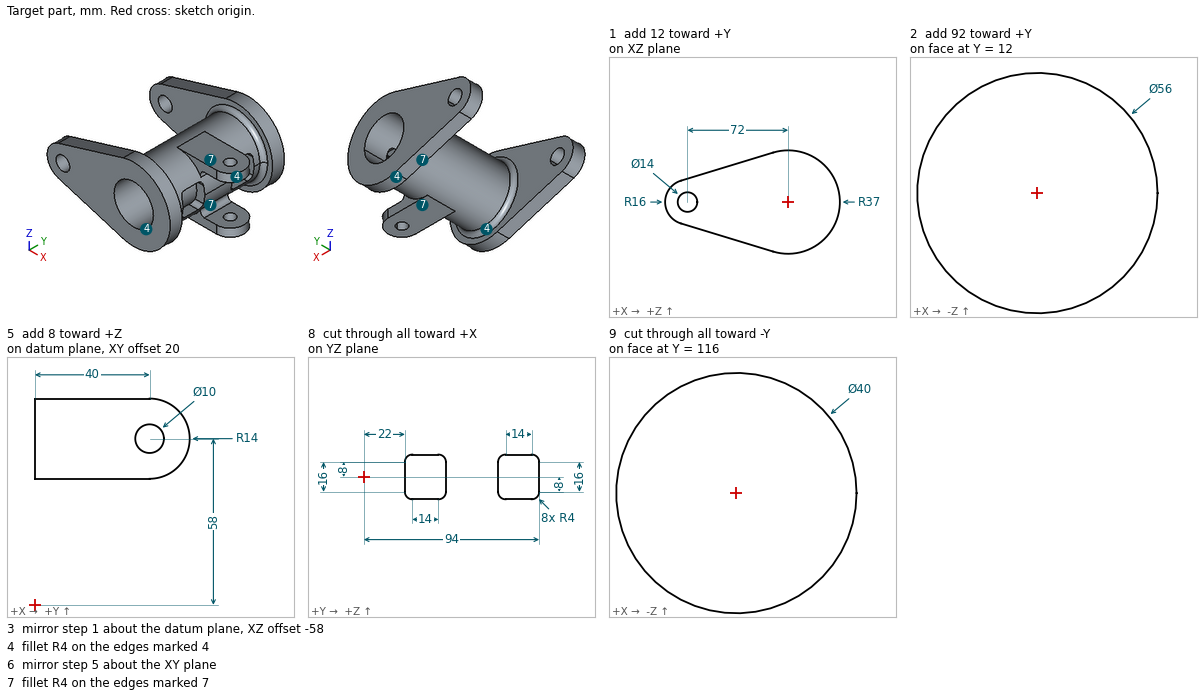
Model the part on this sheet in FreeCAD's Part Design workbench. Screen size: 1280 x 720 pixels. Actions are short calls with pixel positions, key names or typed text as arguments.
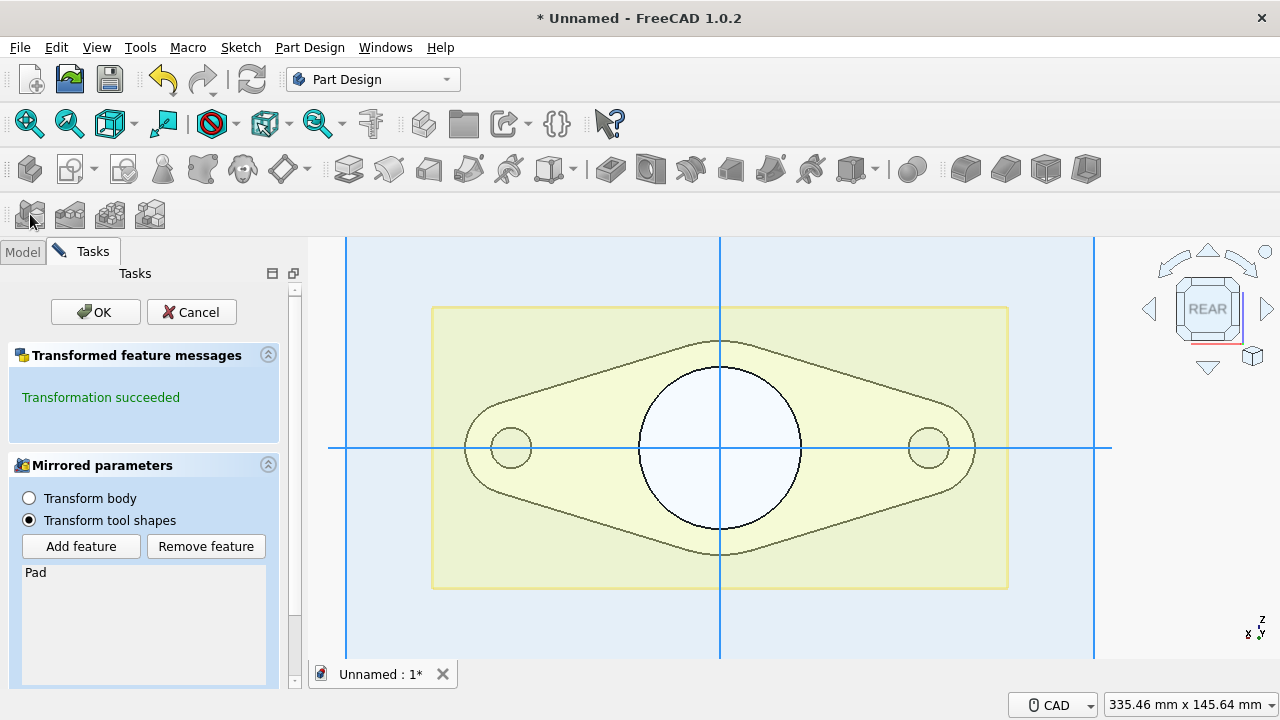
scroll(295, 486, down, 2)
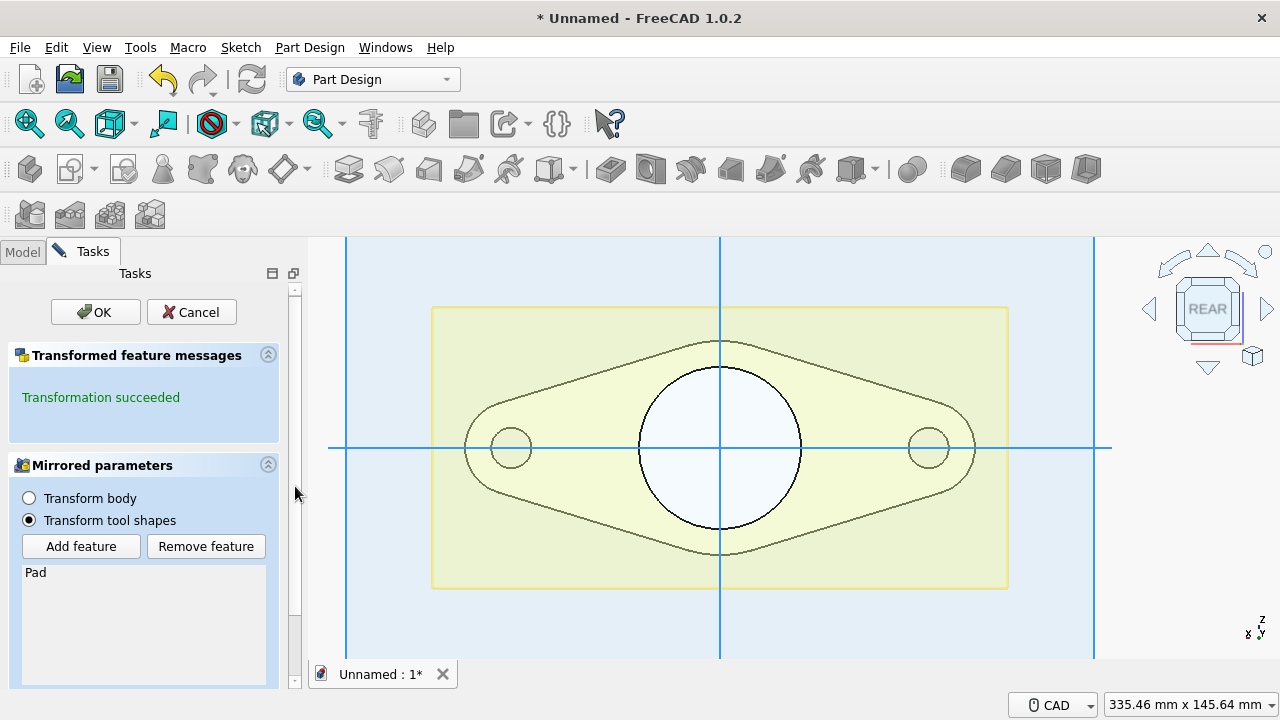
click(184, 628)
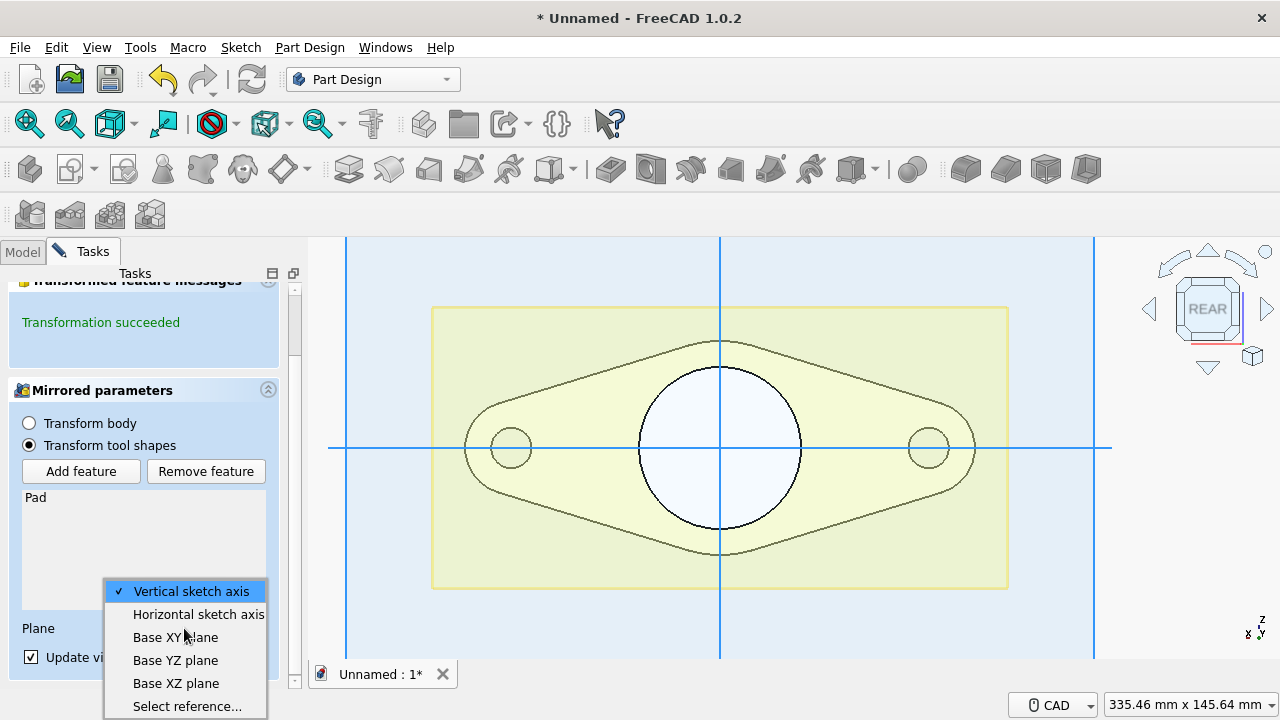
click(184, 706)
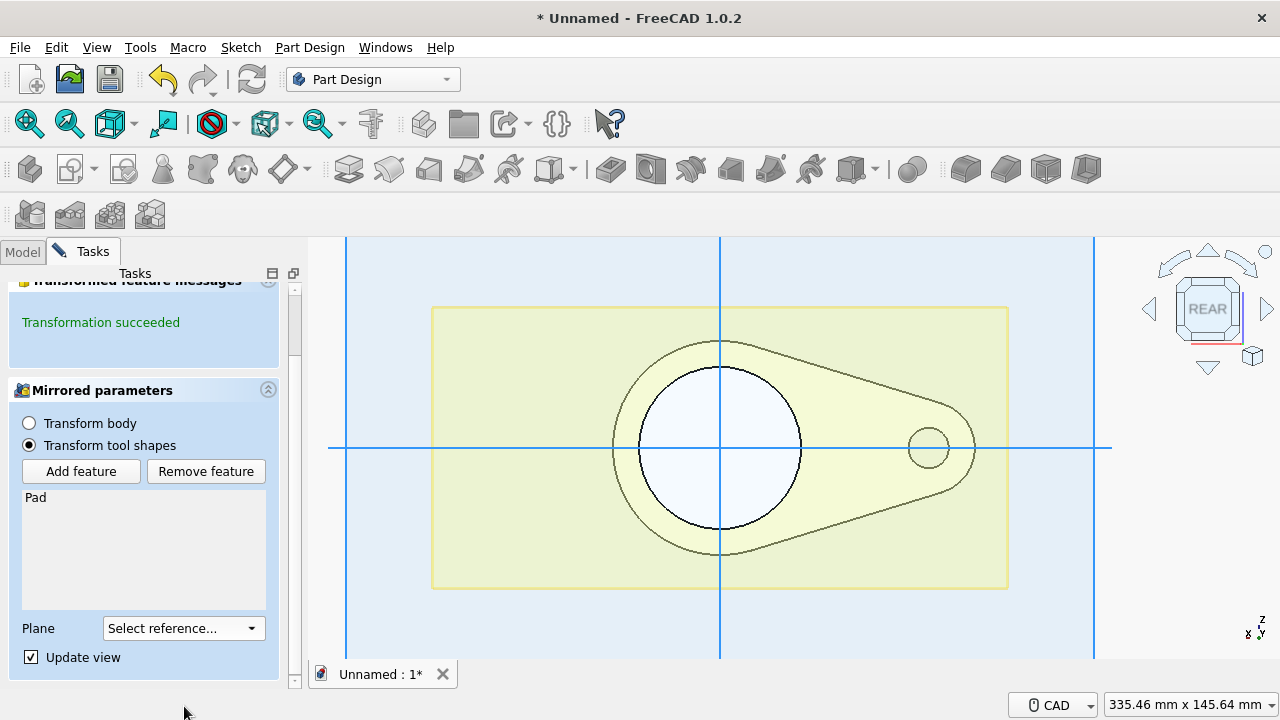
click(23, 251)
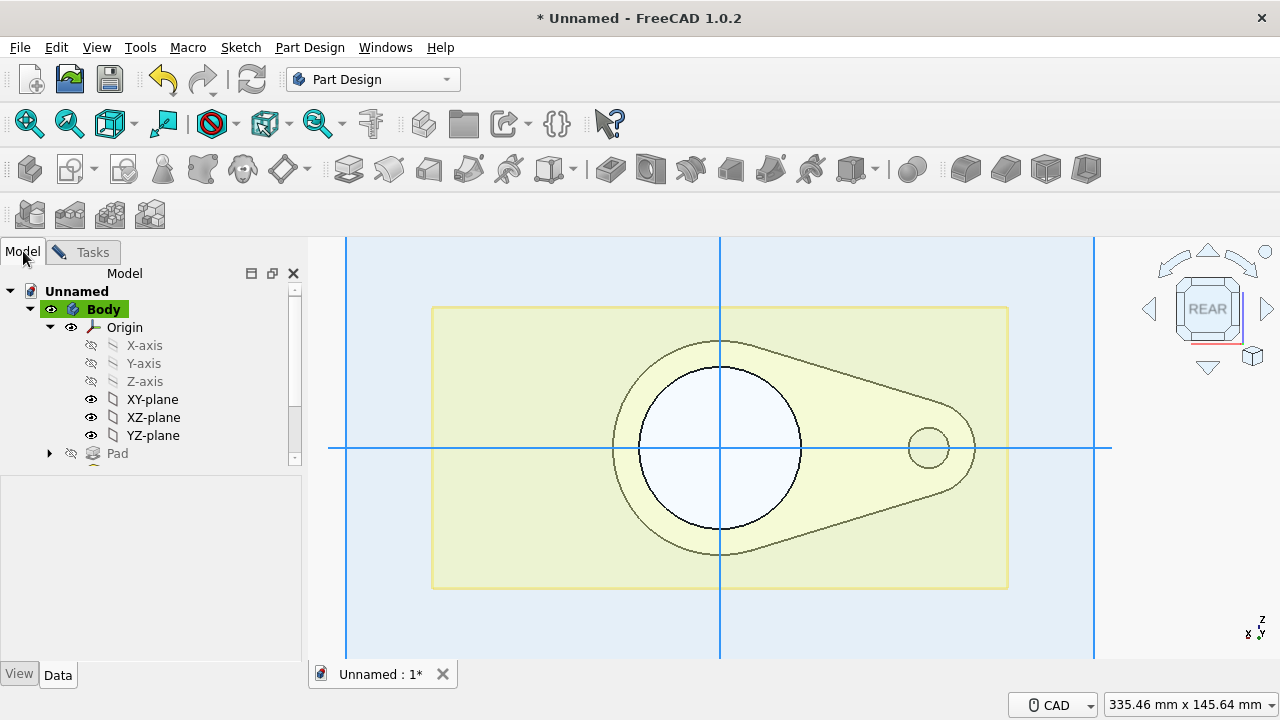
scroll(100, 377, down, 3)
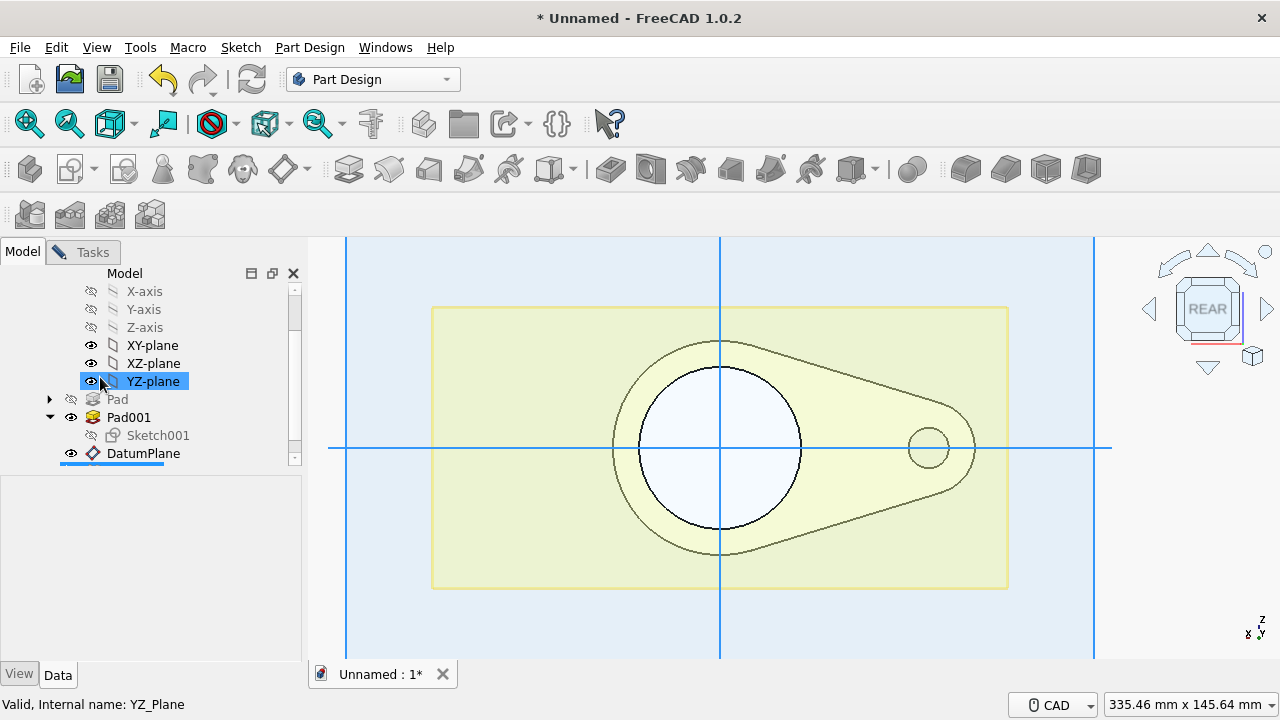
click(116, 435)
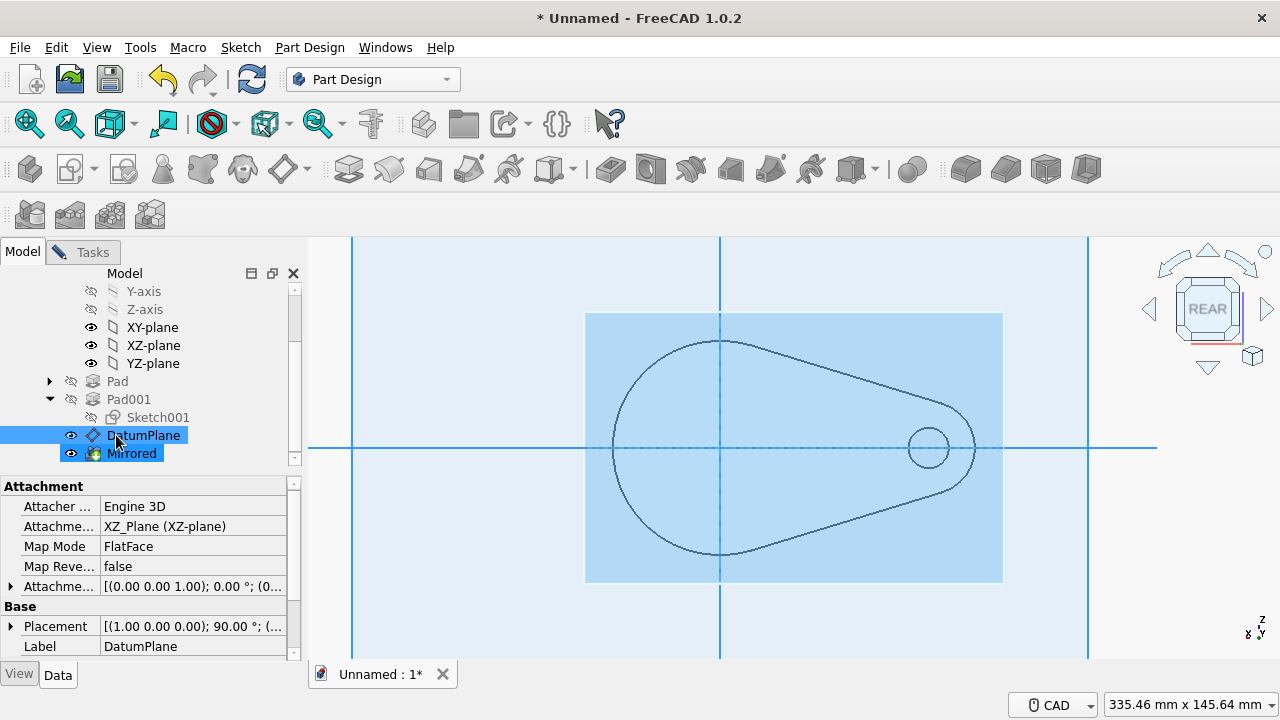
click(84, 251)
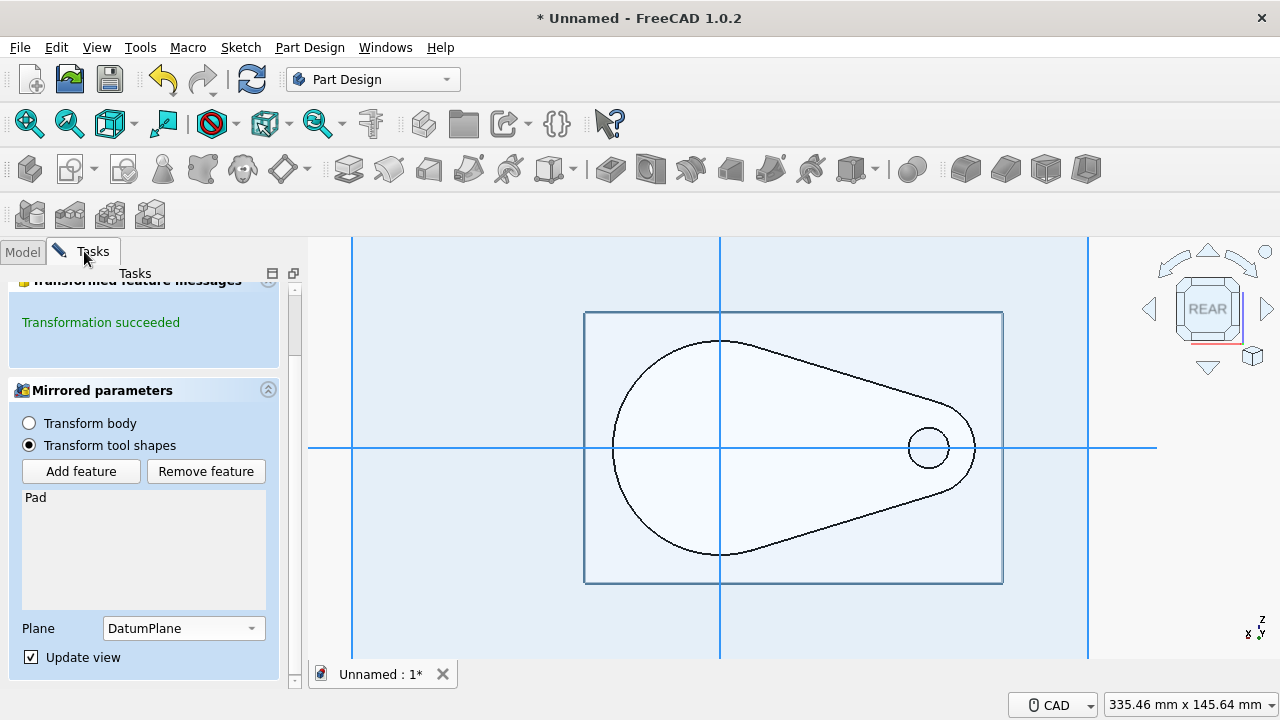
scroll(295, 486, up, 2)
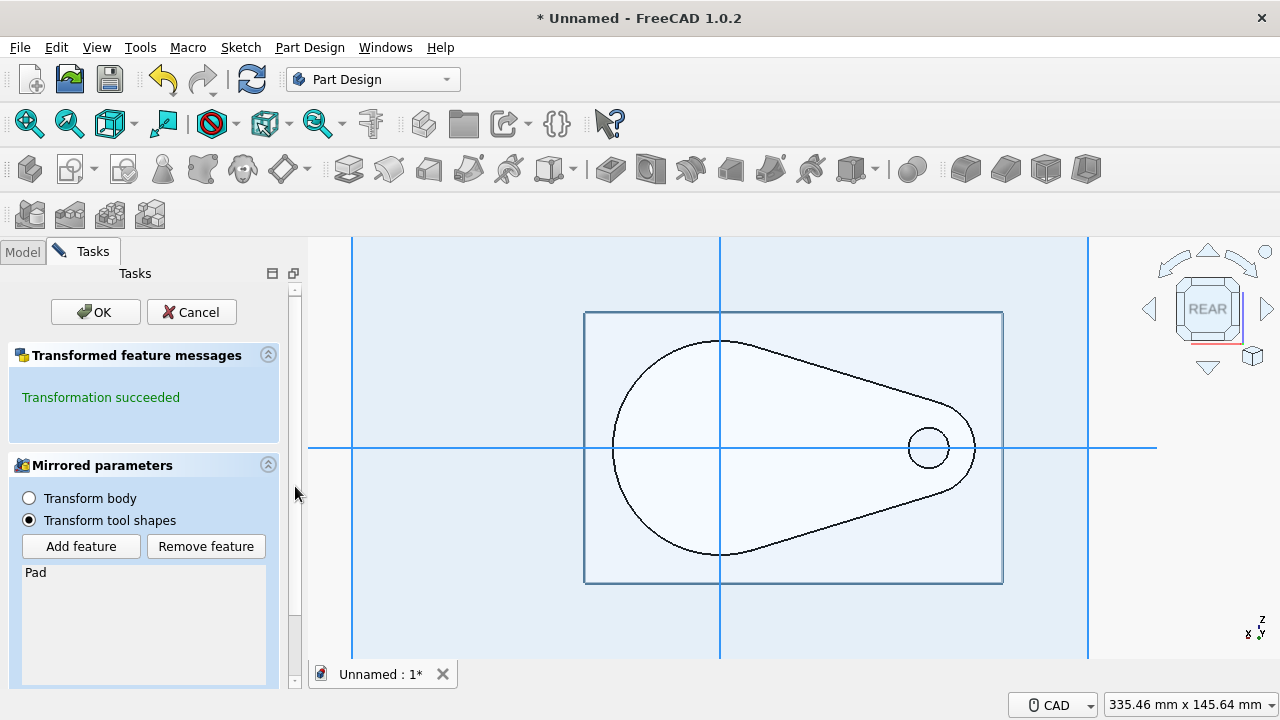
click(96, 312)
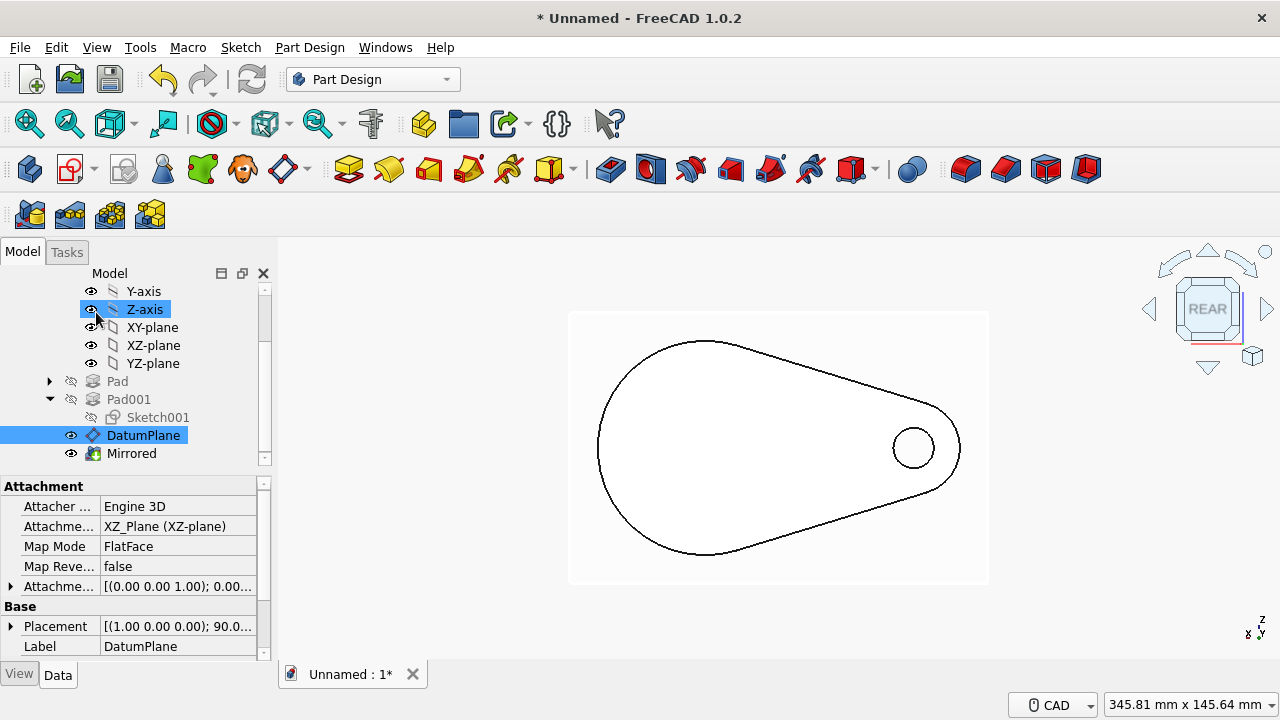
click(116, 435)
key(space)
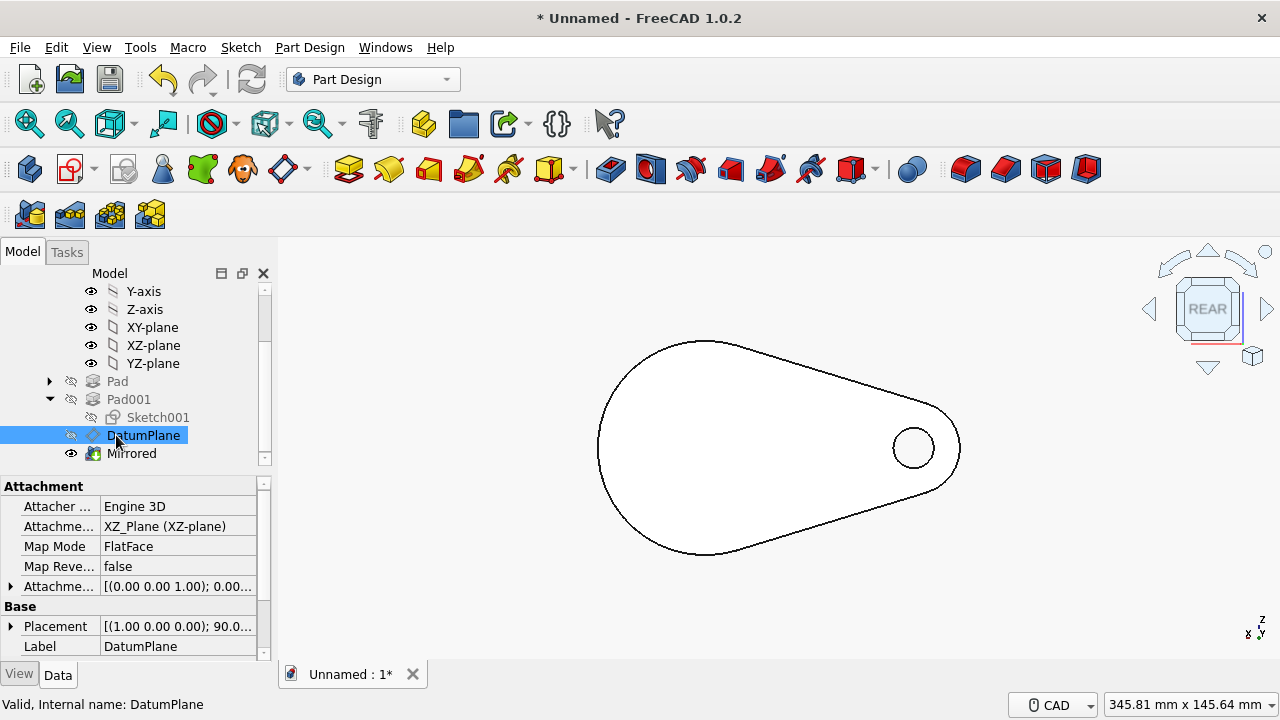
key(0)